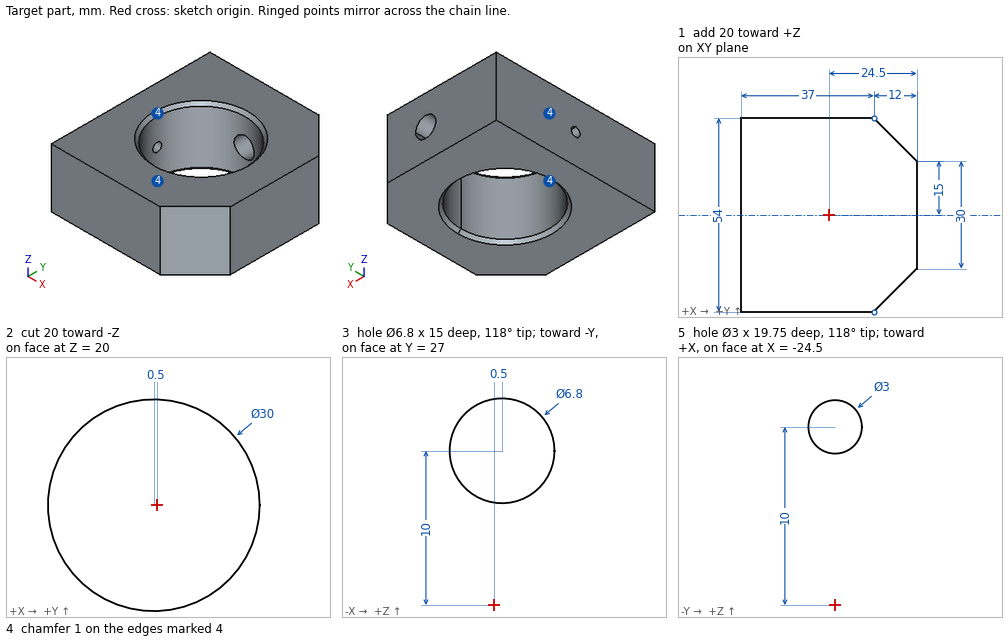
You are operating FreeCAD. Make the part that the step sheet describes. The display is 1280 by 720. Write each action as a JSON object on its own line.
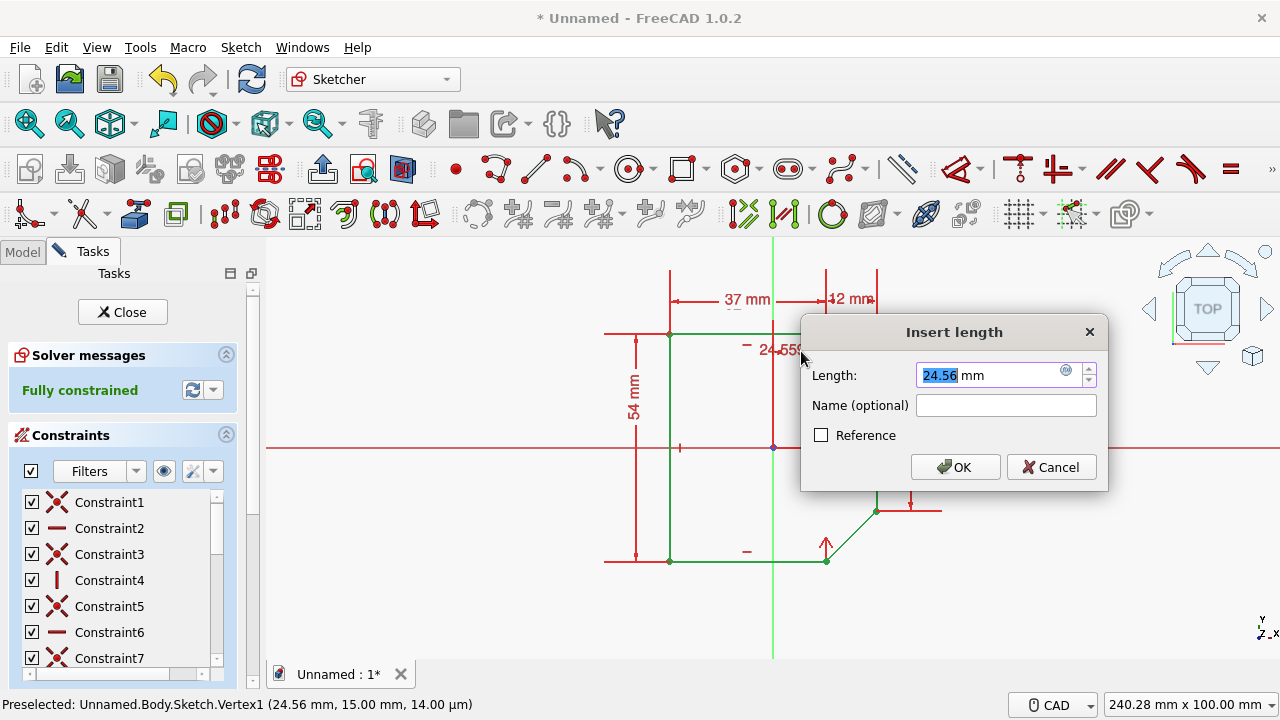
{"action": "type", "text": "24.5"}
{"action": "key", "text": "Return"}
{"action": "key", "text": "Escape"}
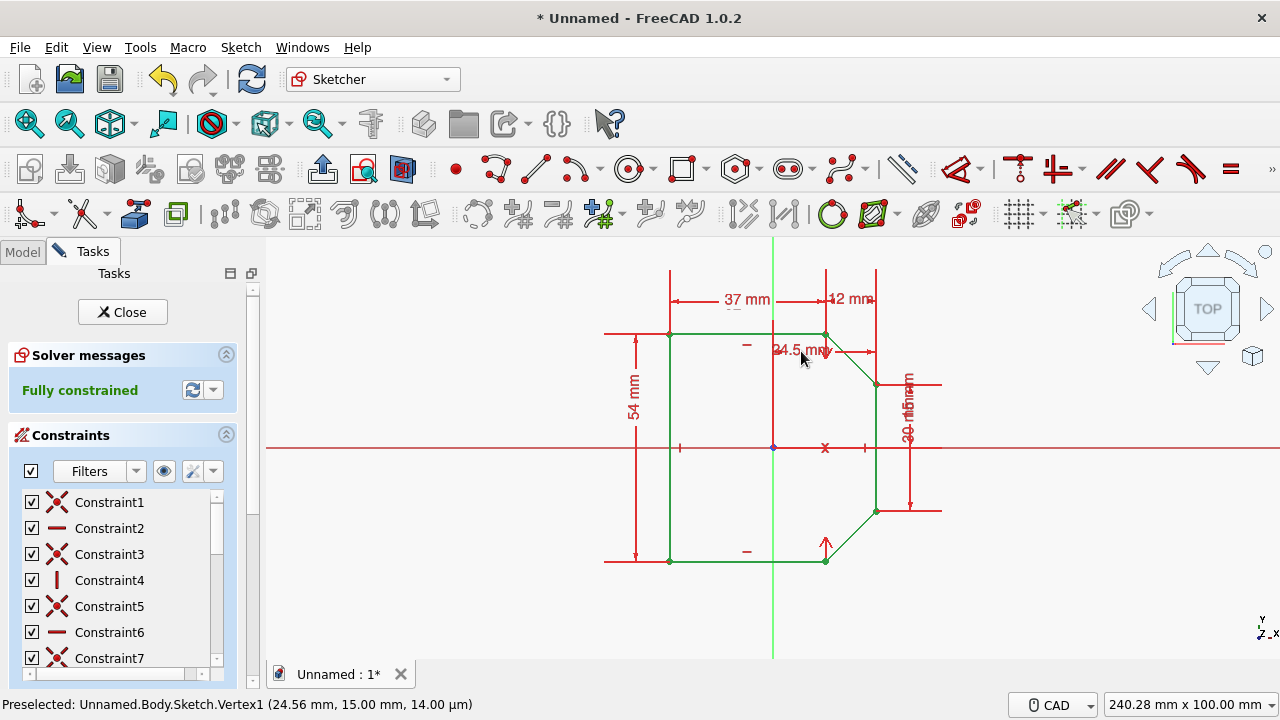
{"action": "left_click", "coordinate": [123, 312]}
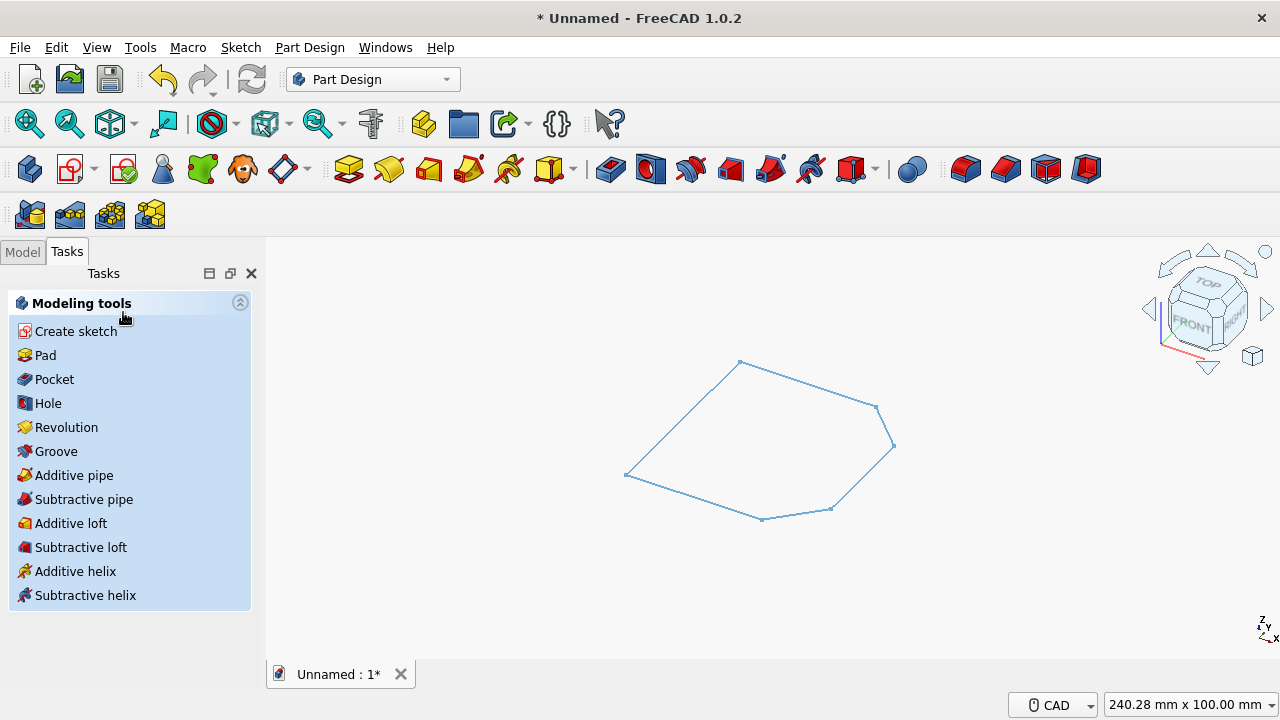
{"action": "left_click", "coordinate": [350, 170]}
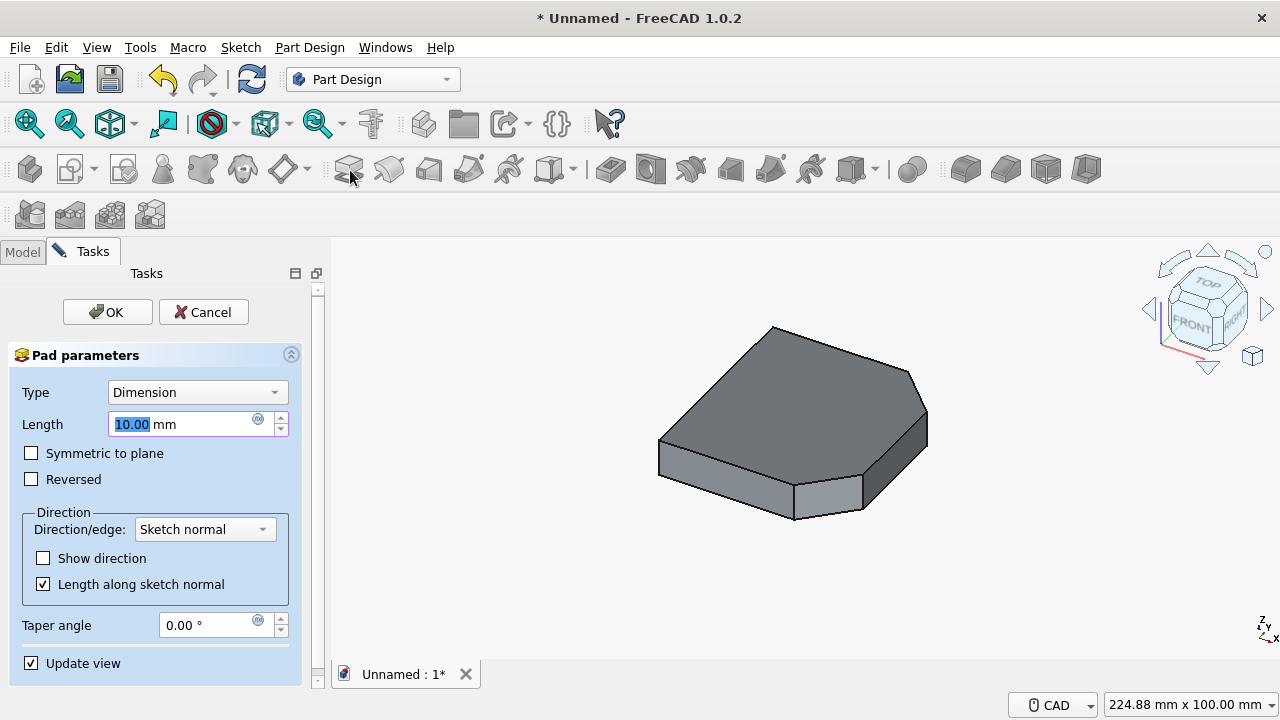
{"action": "type", "text": "20"}
{"action": "key", "text": "Tab"}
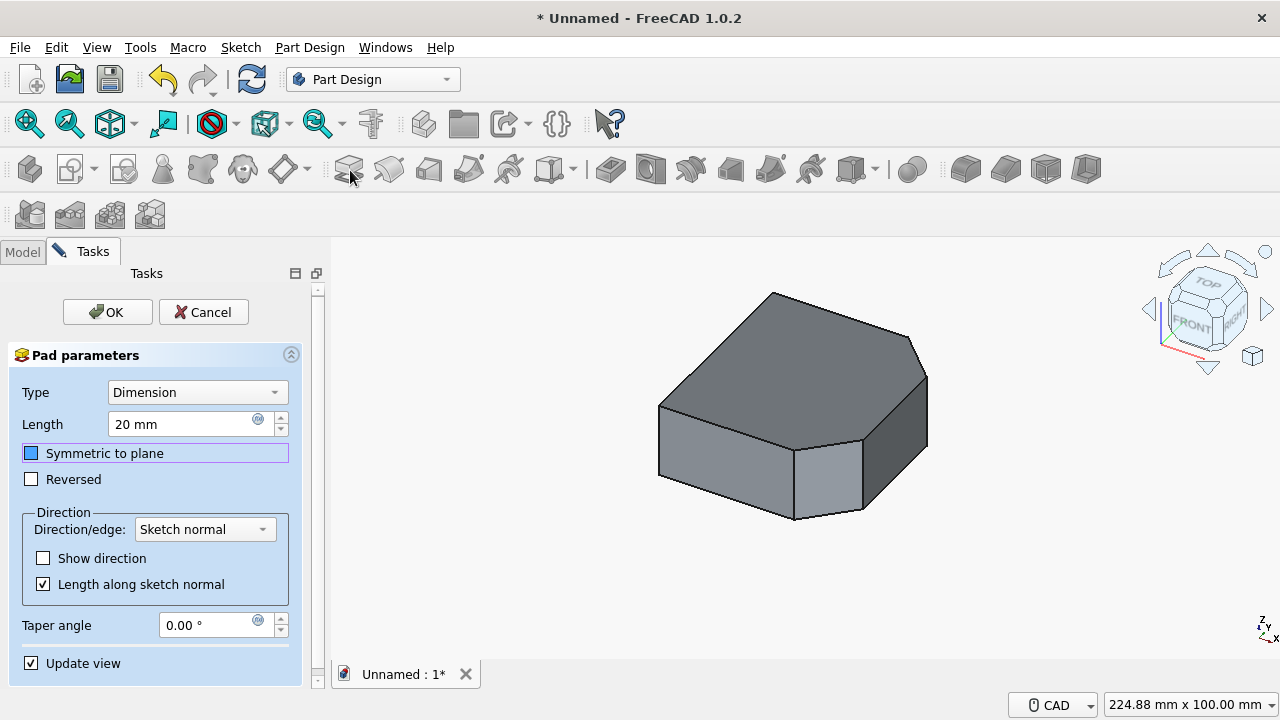
{"action": "left_click", "coordinate": [108, 312]}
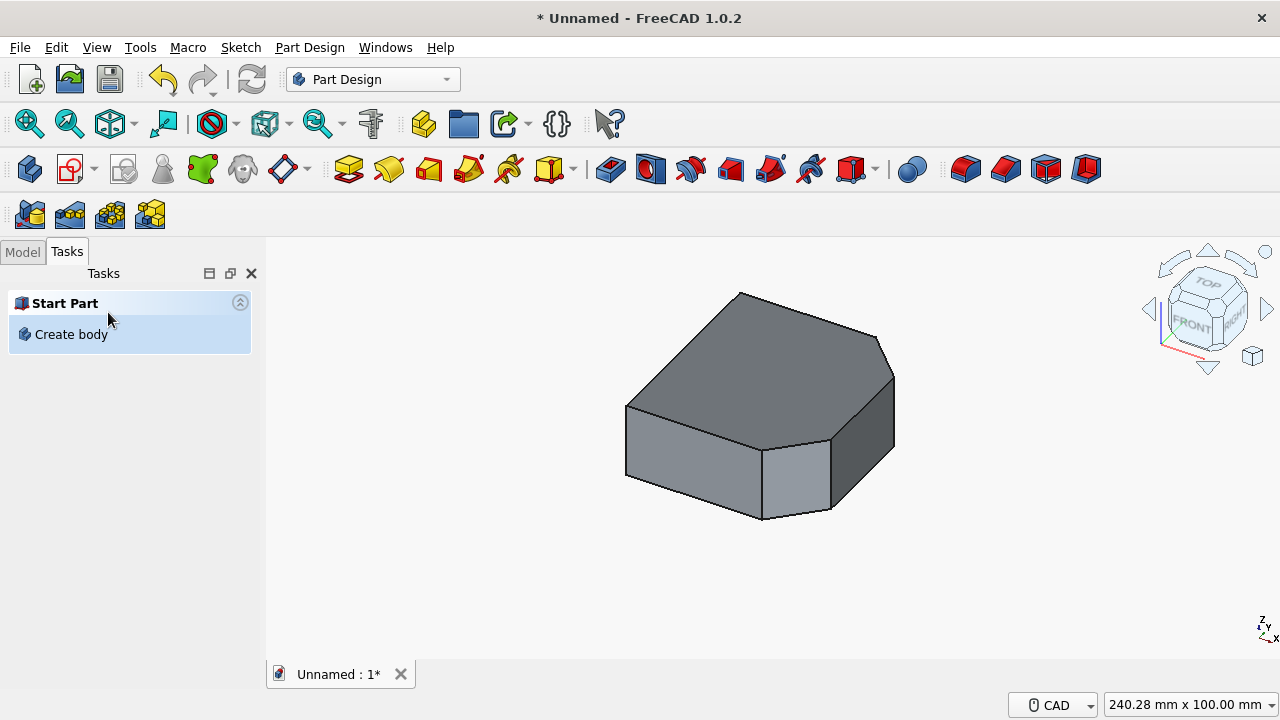
{"action": "left_click", "coordinate": [773, 378]}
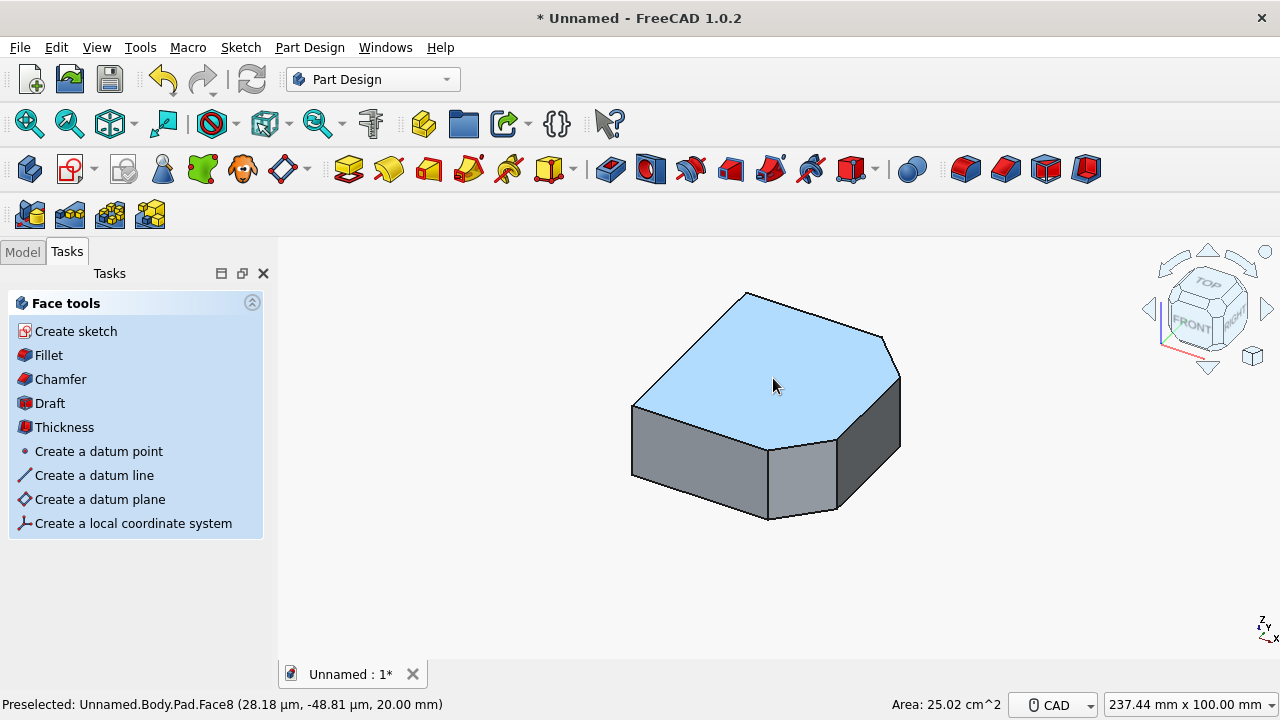
{"action": "left_click", "coordinate": [70, 170]}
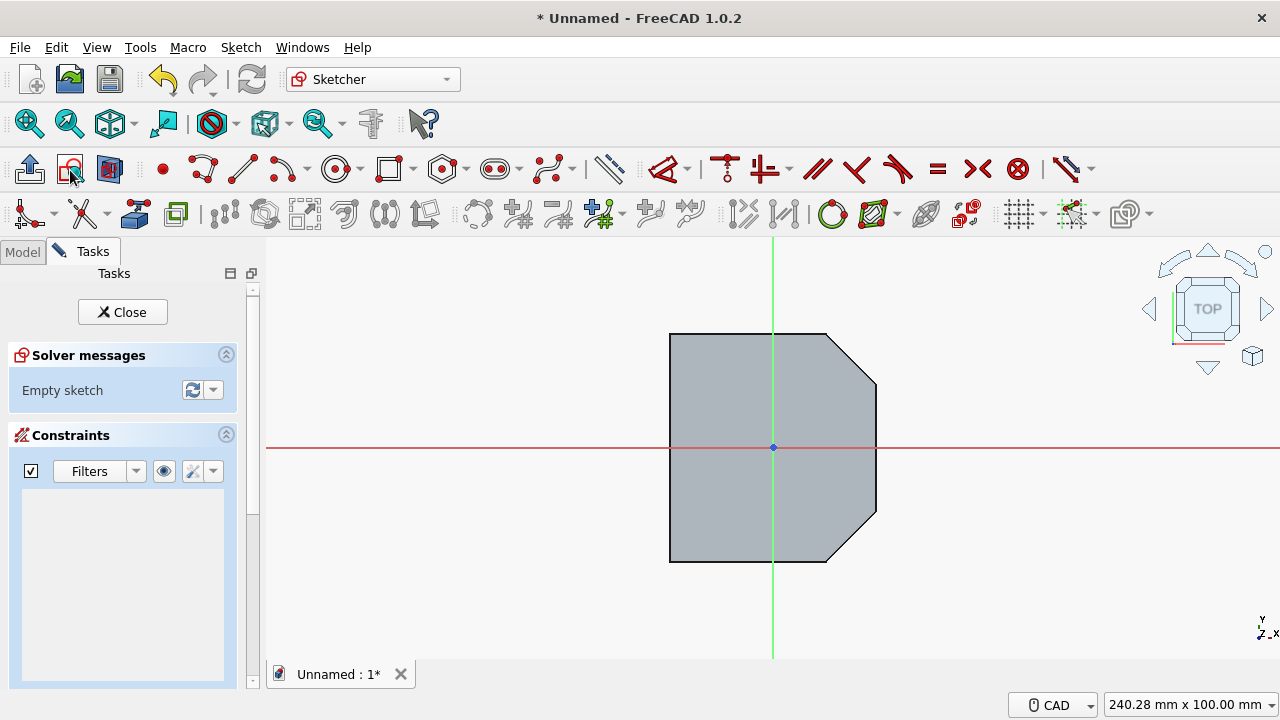
{"action": "scroll", "coordinate": [825, 448], "scroll_direction": "up", "scroll_amount": 4}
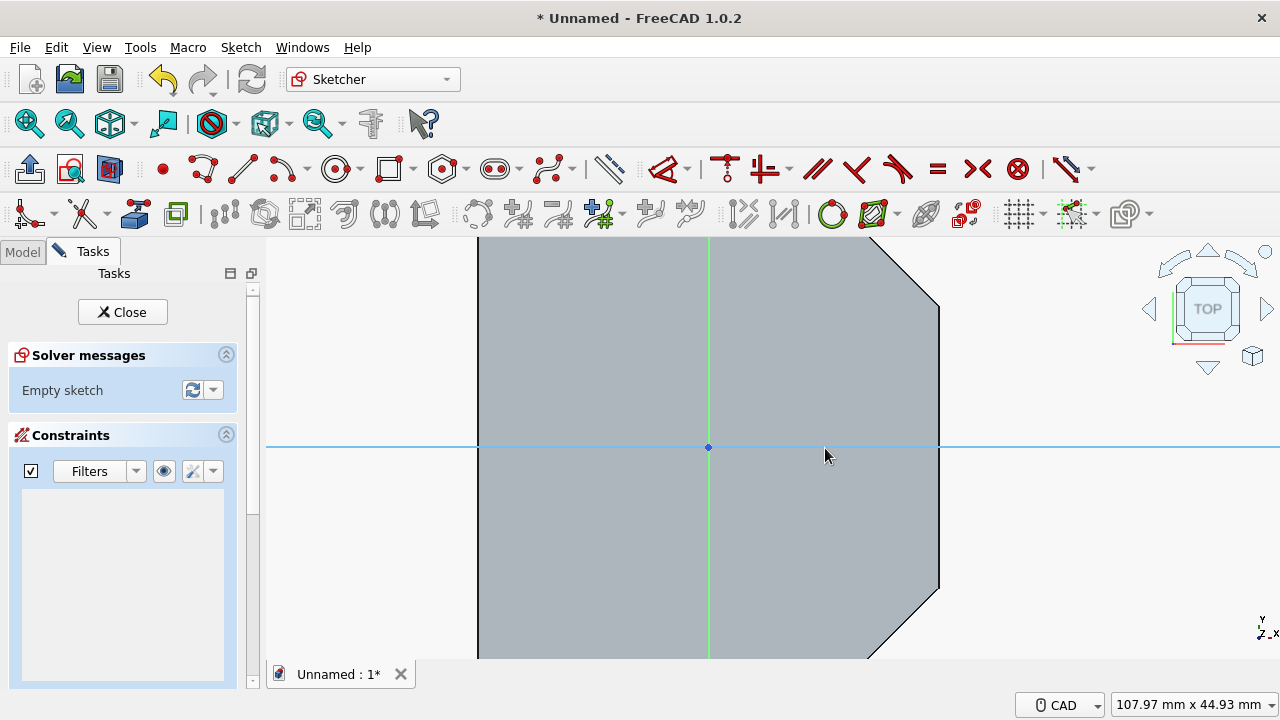
{"action": "key", "text": "g c"}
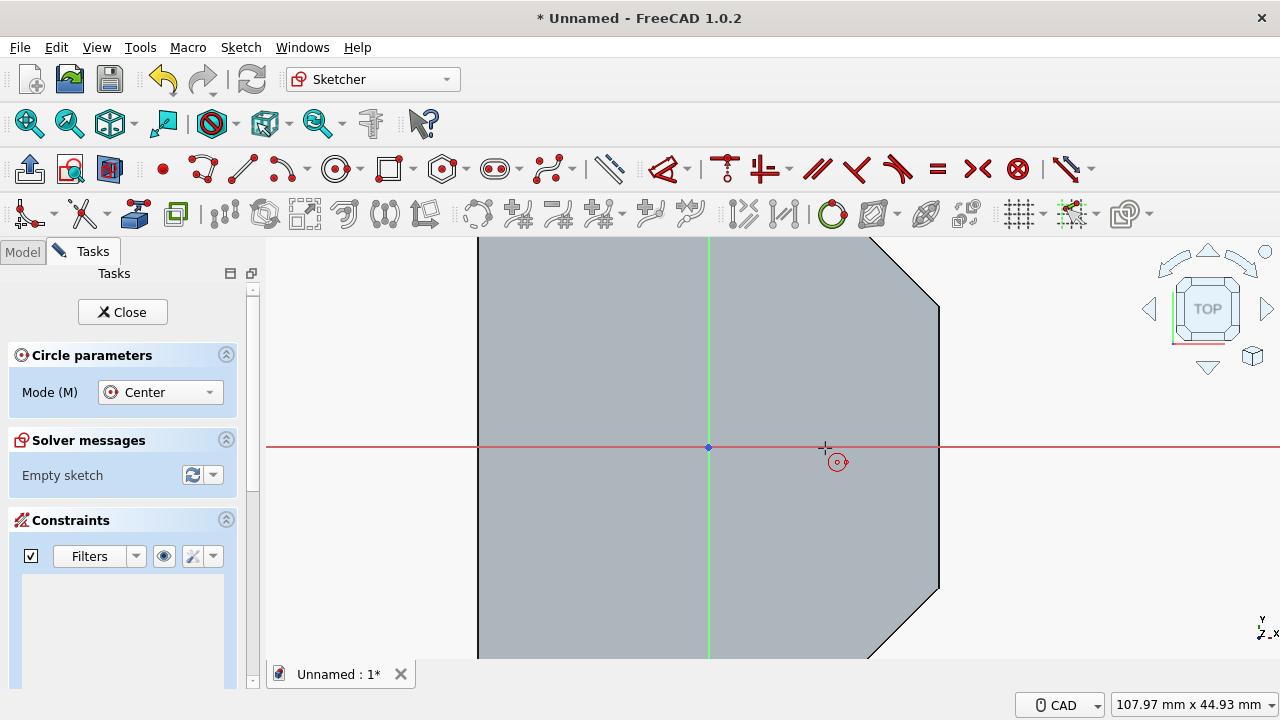
{"action": "scroll", "coordinate": [704, 447], "scroll_direction": "up", "scroll_amount": 7}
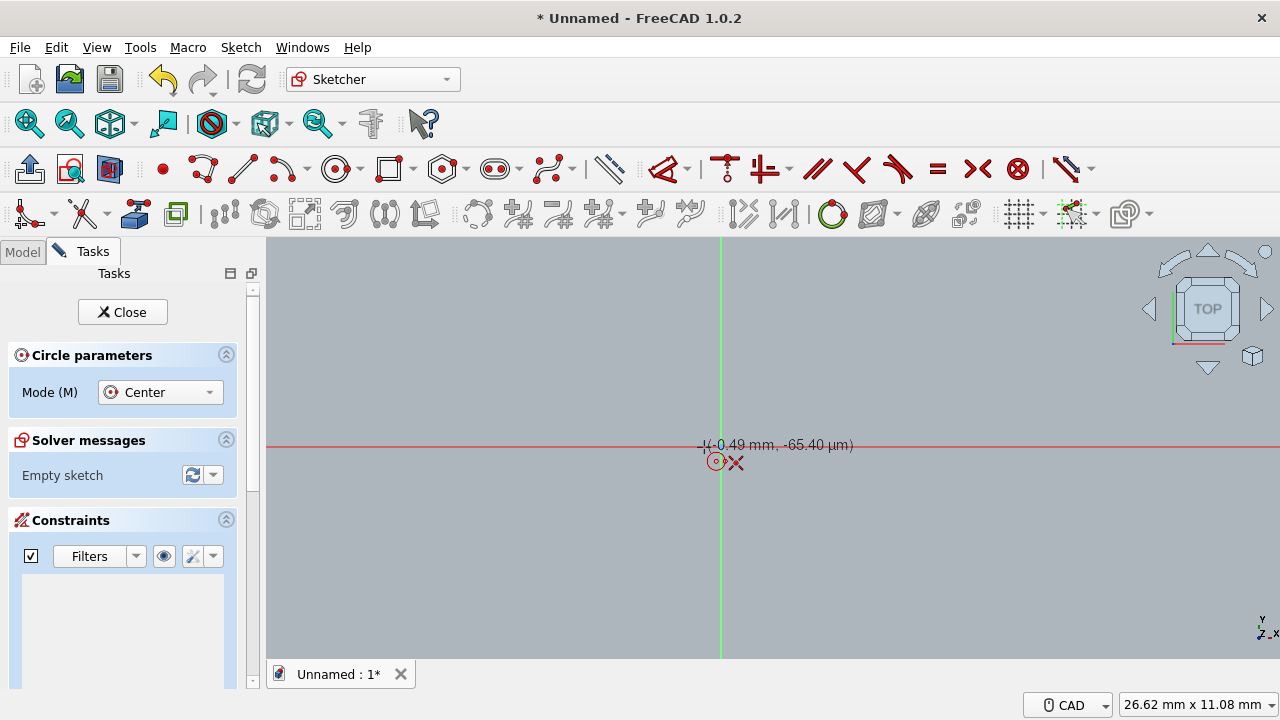
{"action": "left_click", "coordinate": [702, 447]}